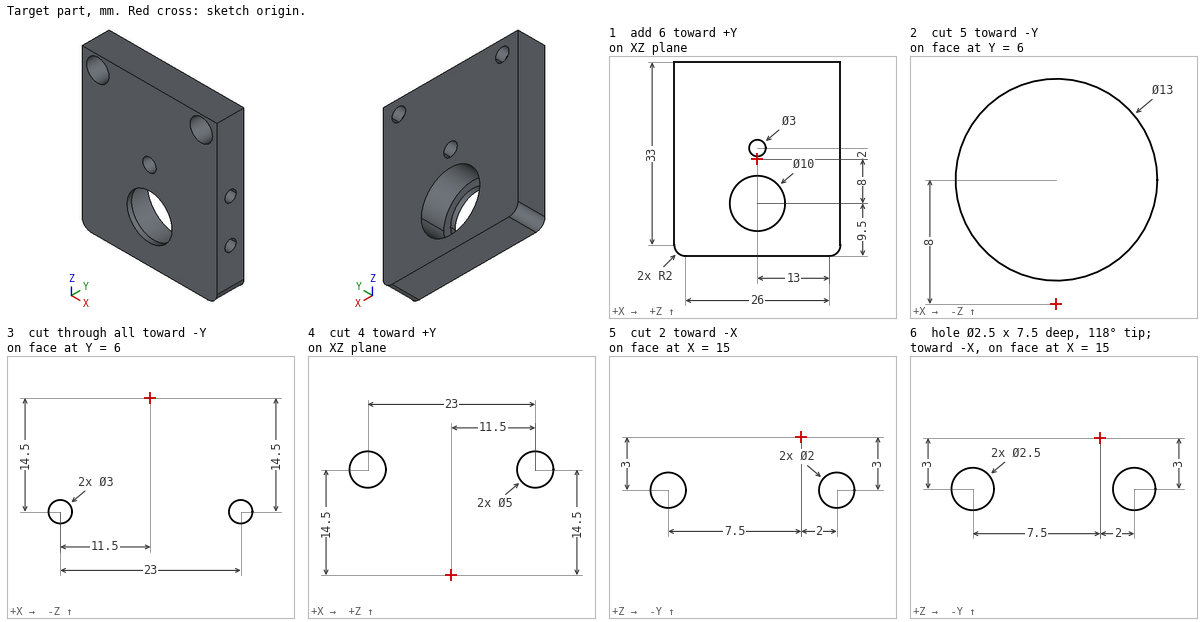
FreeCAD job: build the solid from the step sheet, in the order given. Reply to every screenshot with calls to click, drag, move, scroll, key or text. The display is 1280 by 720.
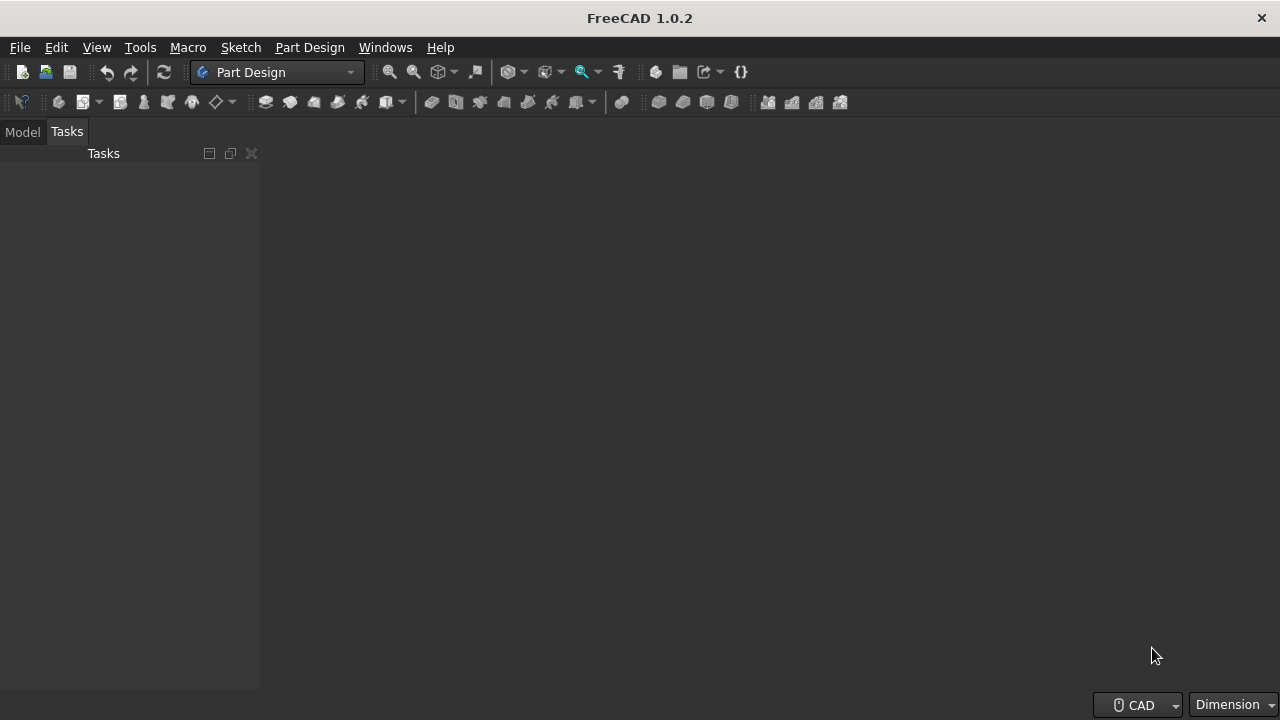
key(ctrl+n)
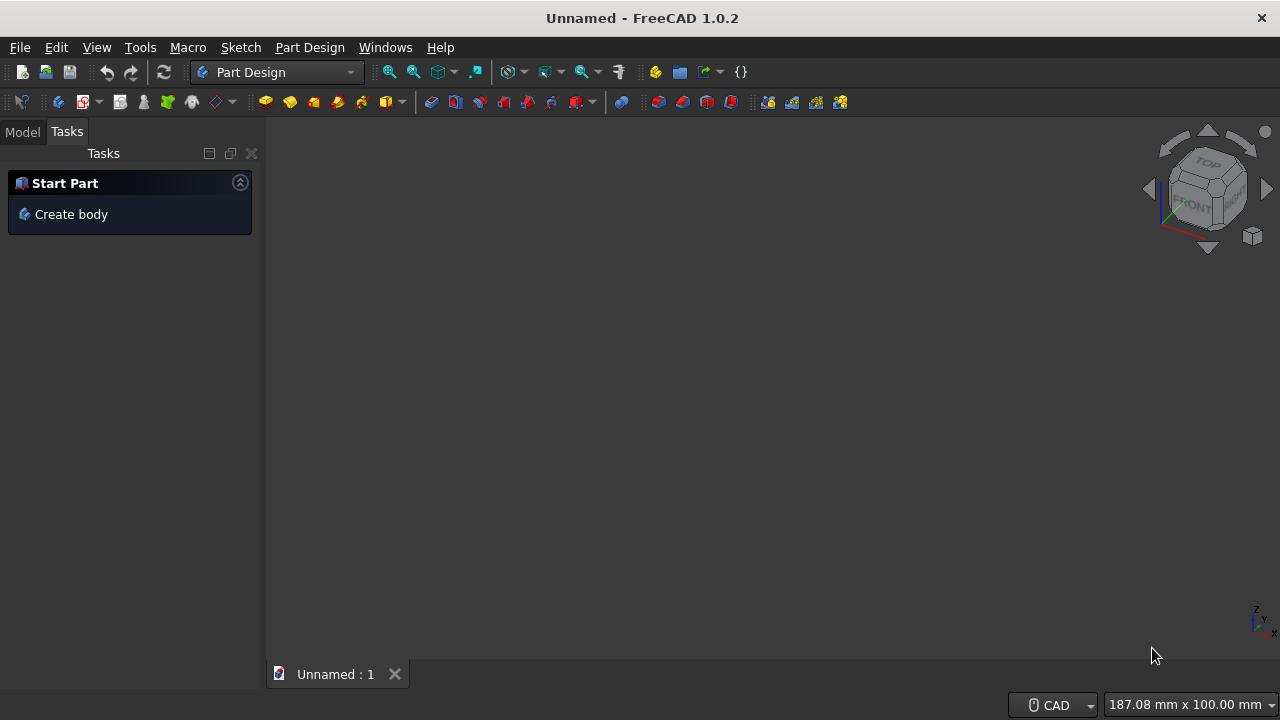
click(84, 102)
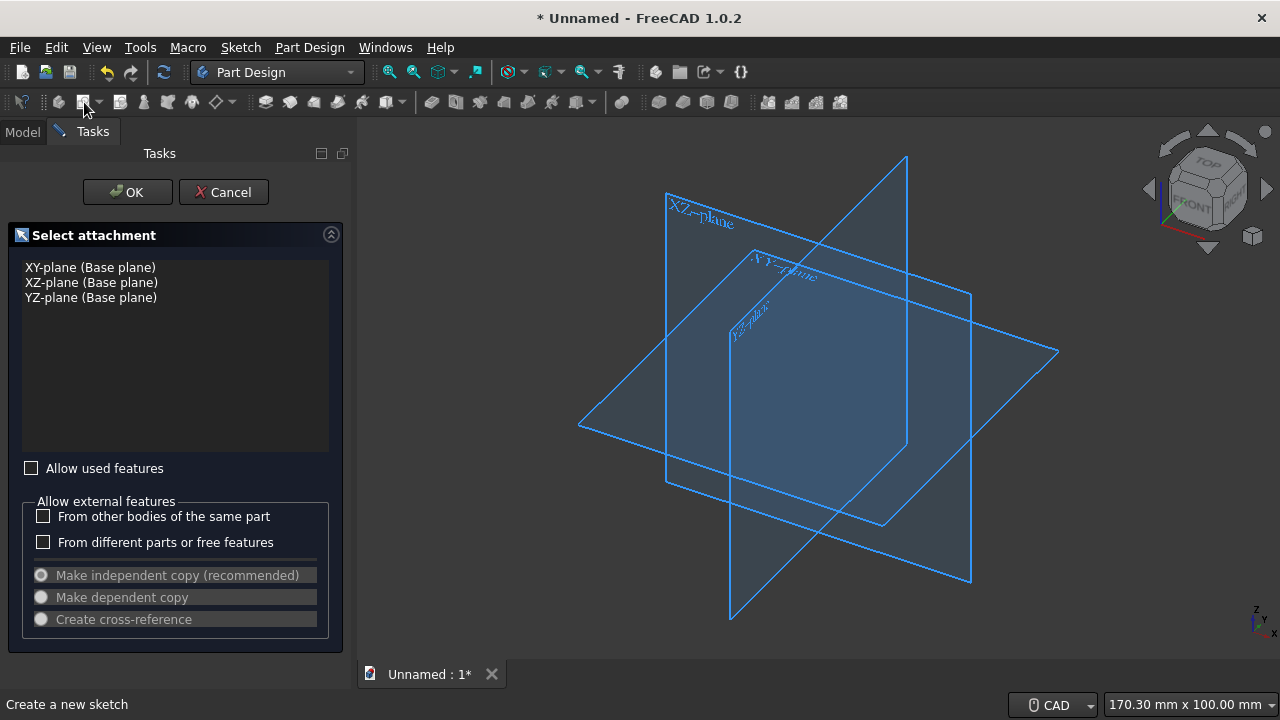
click(82, 282)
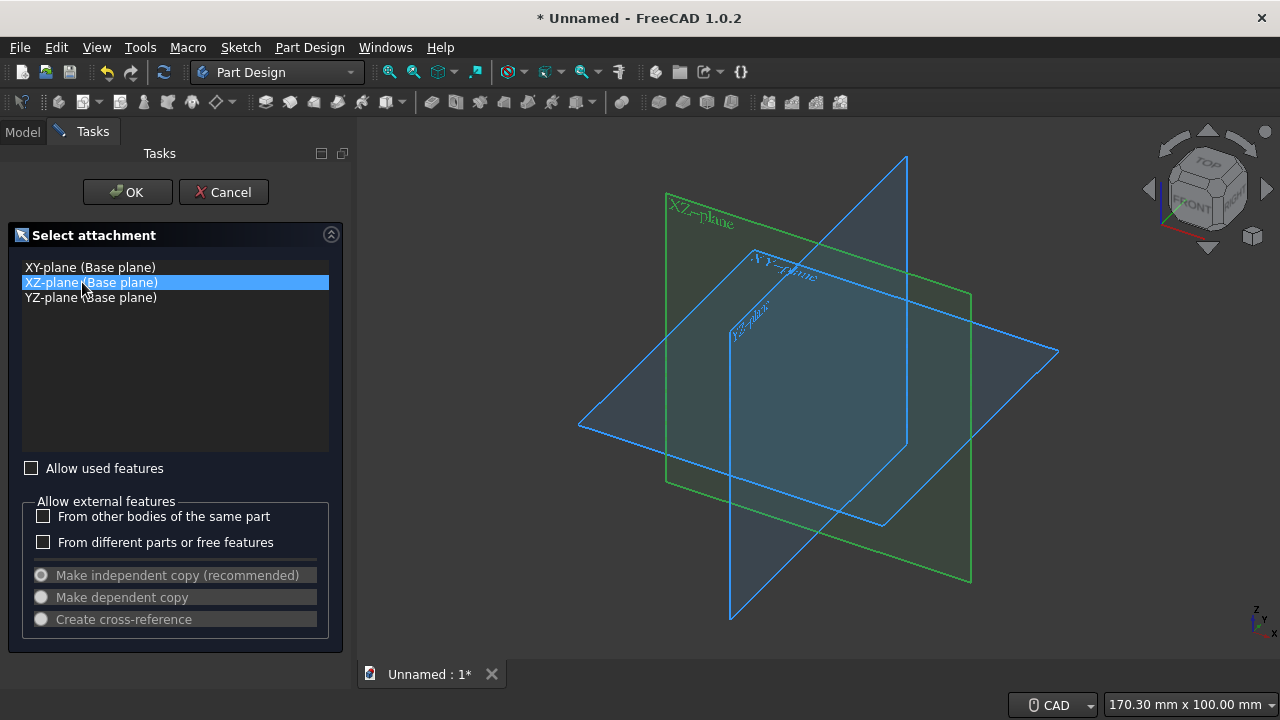
click(128, 192)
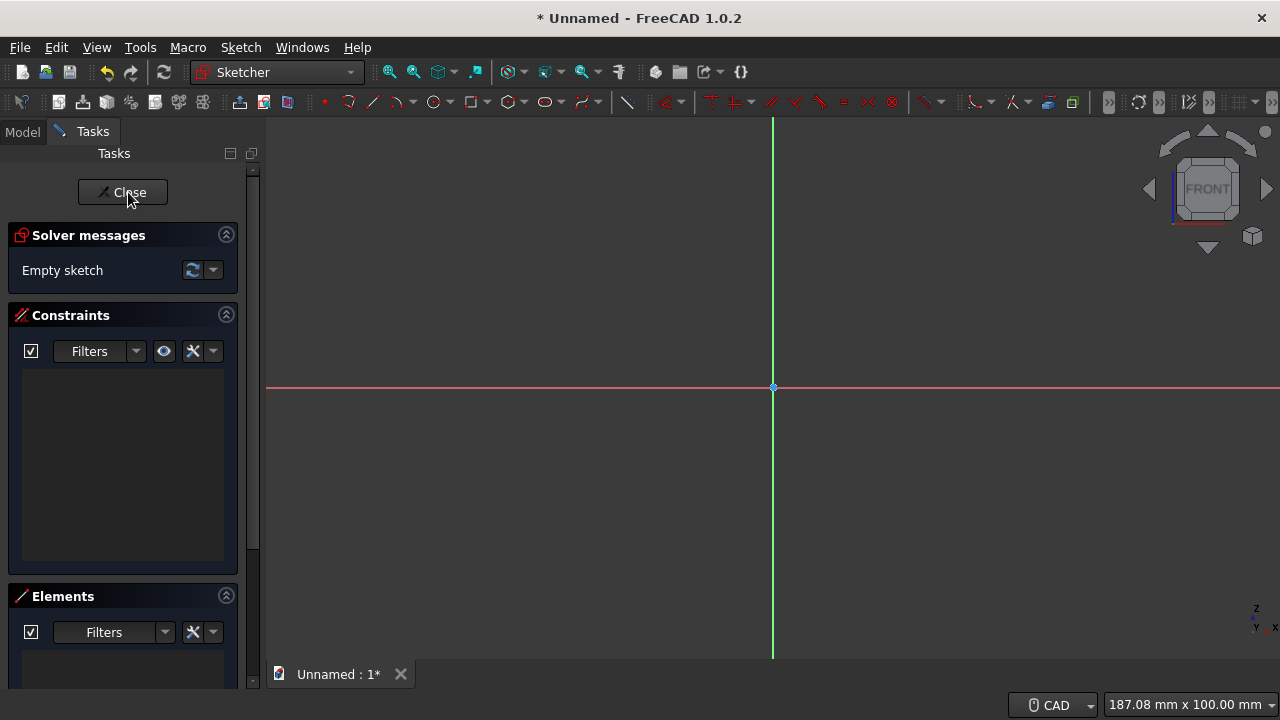
scroll(856, 388, up, 3)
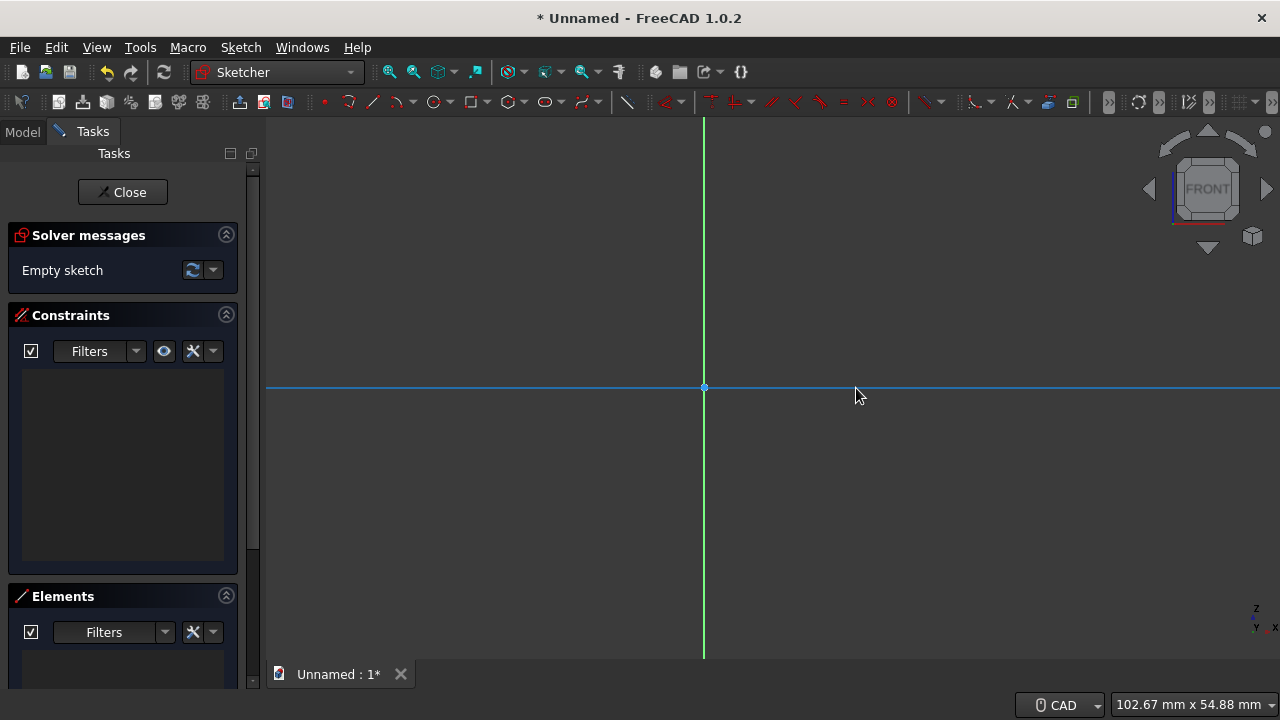
key(g)
key(l)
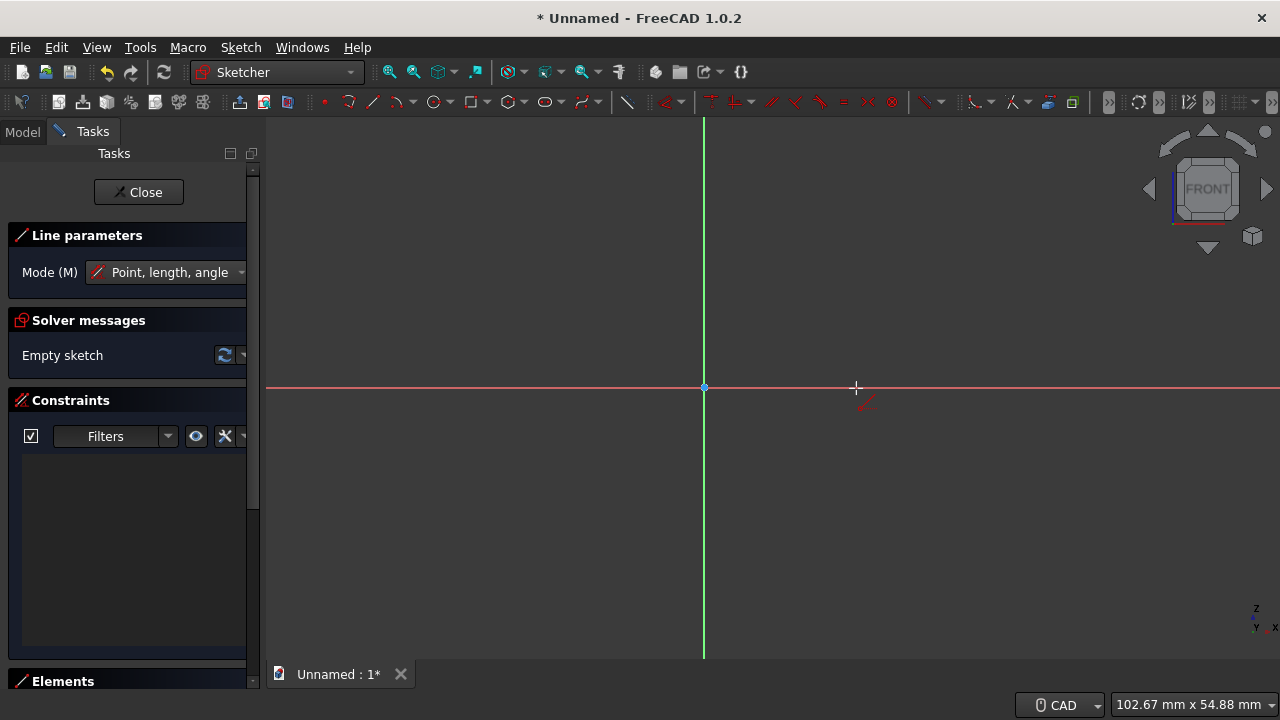
click(833, 560)
click(576, 560)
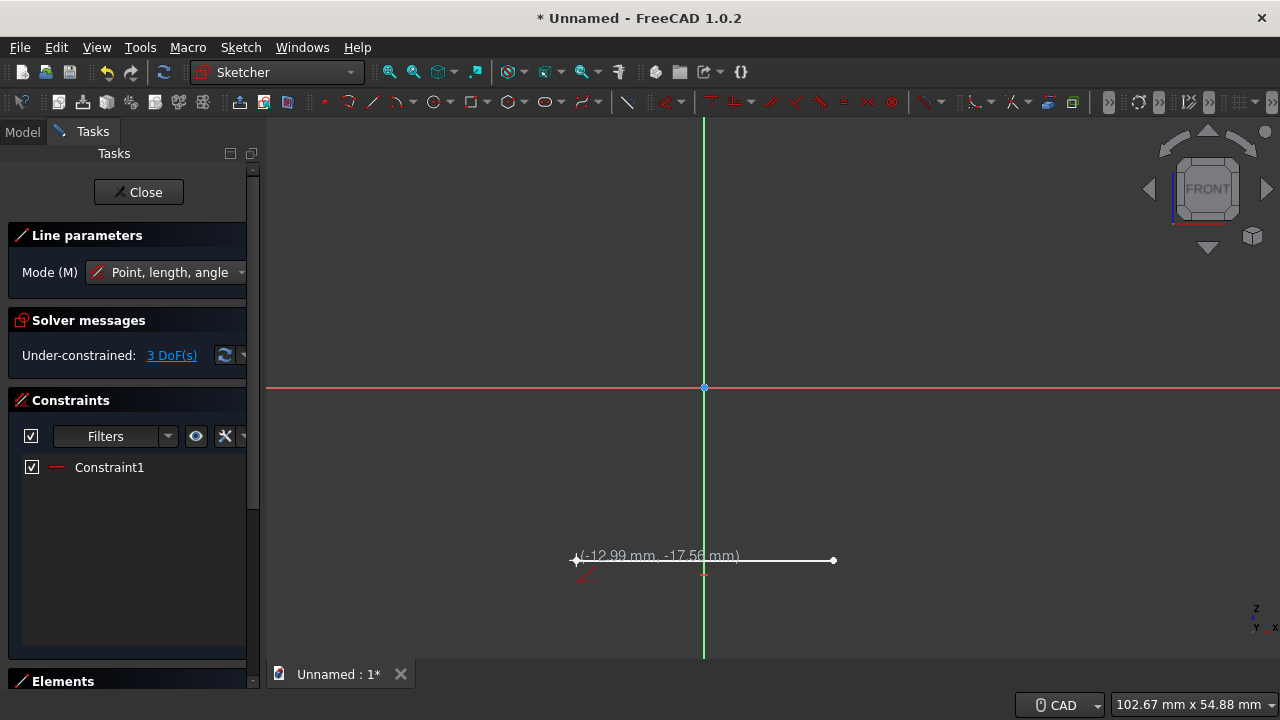
click(350, 102)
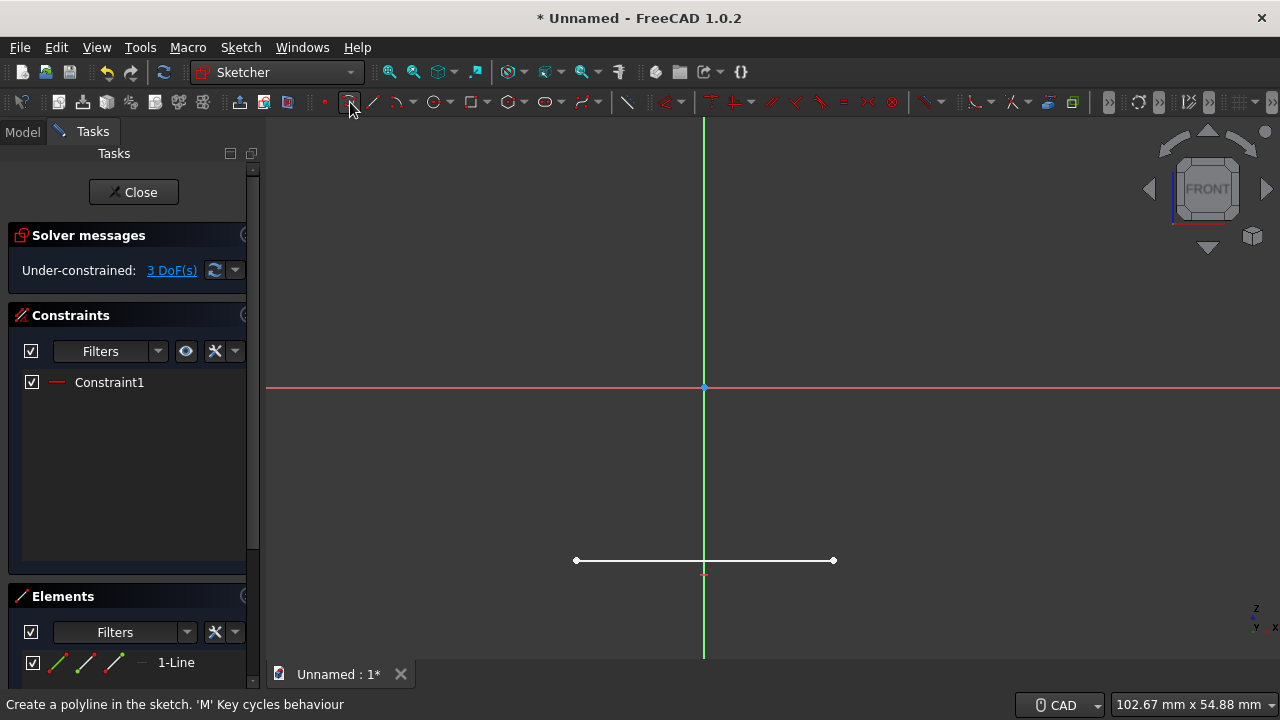
click(556, 541)
click(556, 215)
click(852, 215)
click(852, 541)
right_click(852, 541)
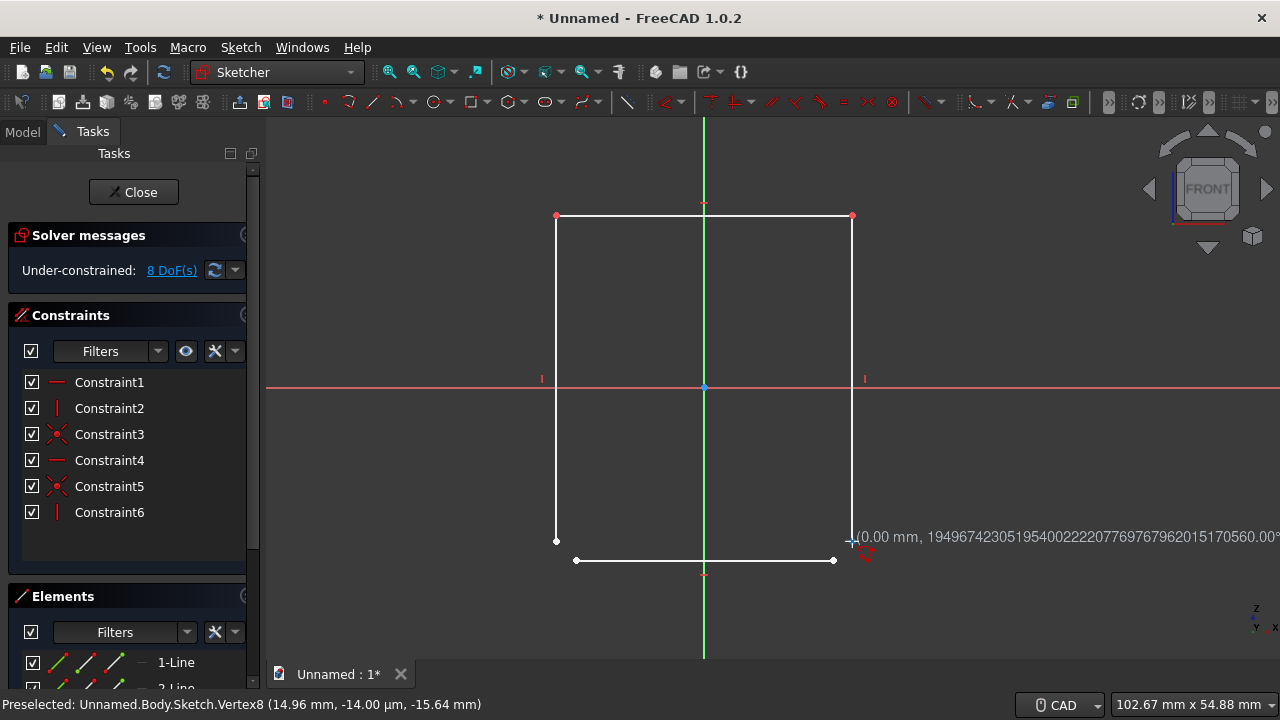
click(416, 102)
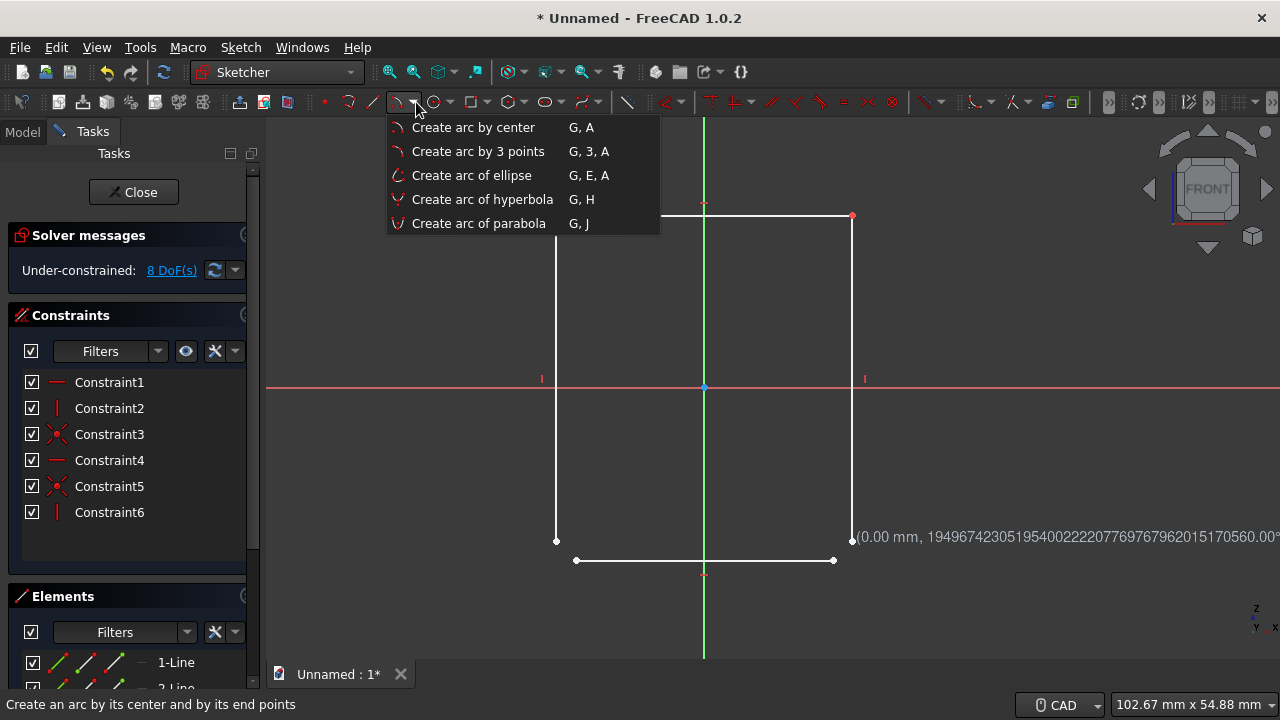
click(524, 151)